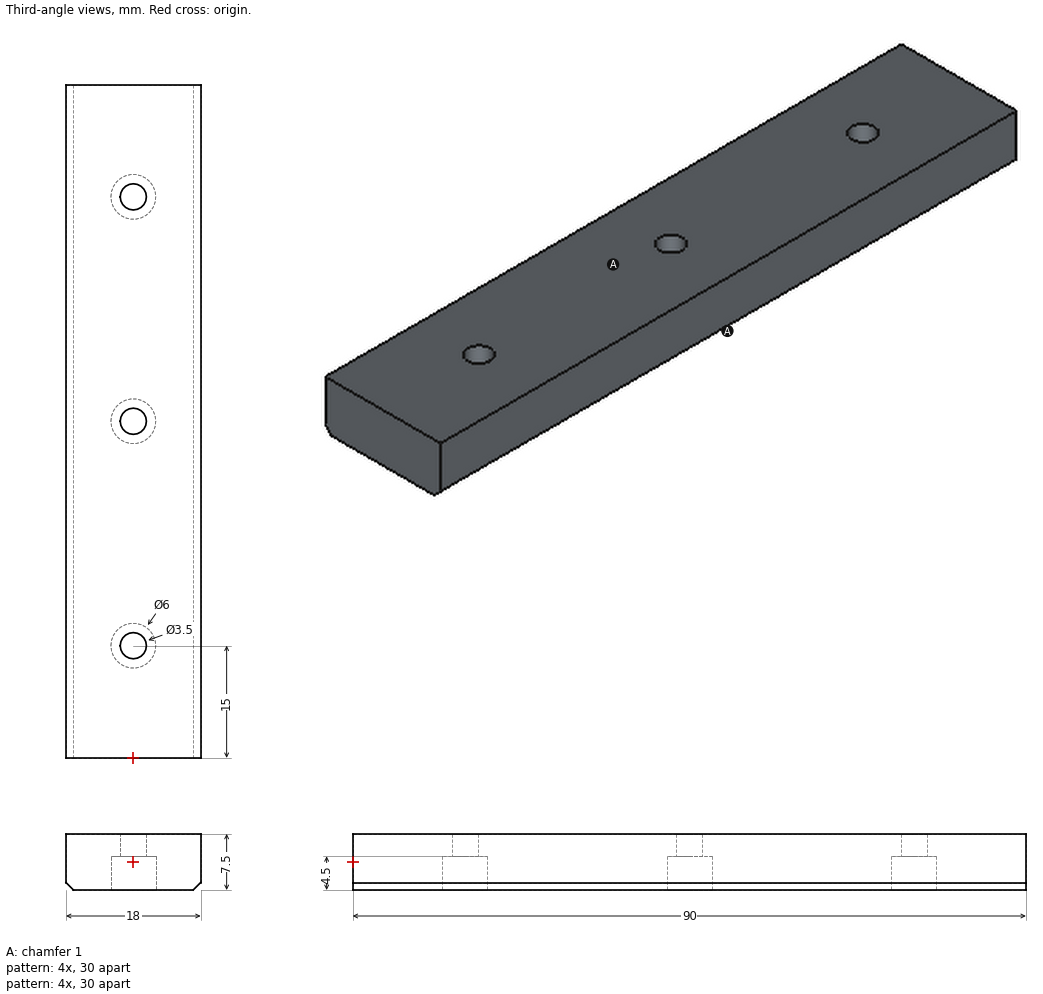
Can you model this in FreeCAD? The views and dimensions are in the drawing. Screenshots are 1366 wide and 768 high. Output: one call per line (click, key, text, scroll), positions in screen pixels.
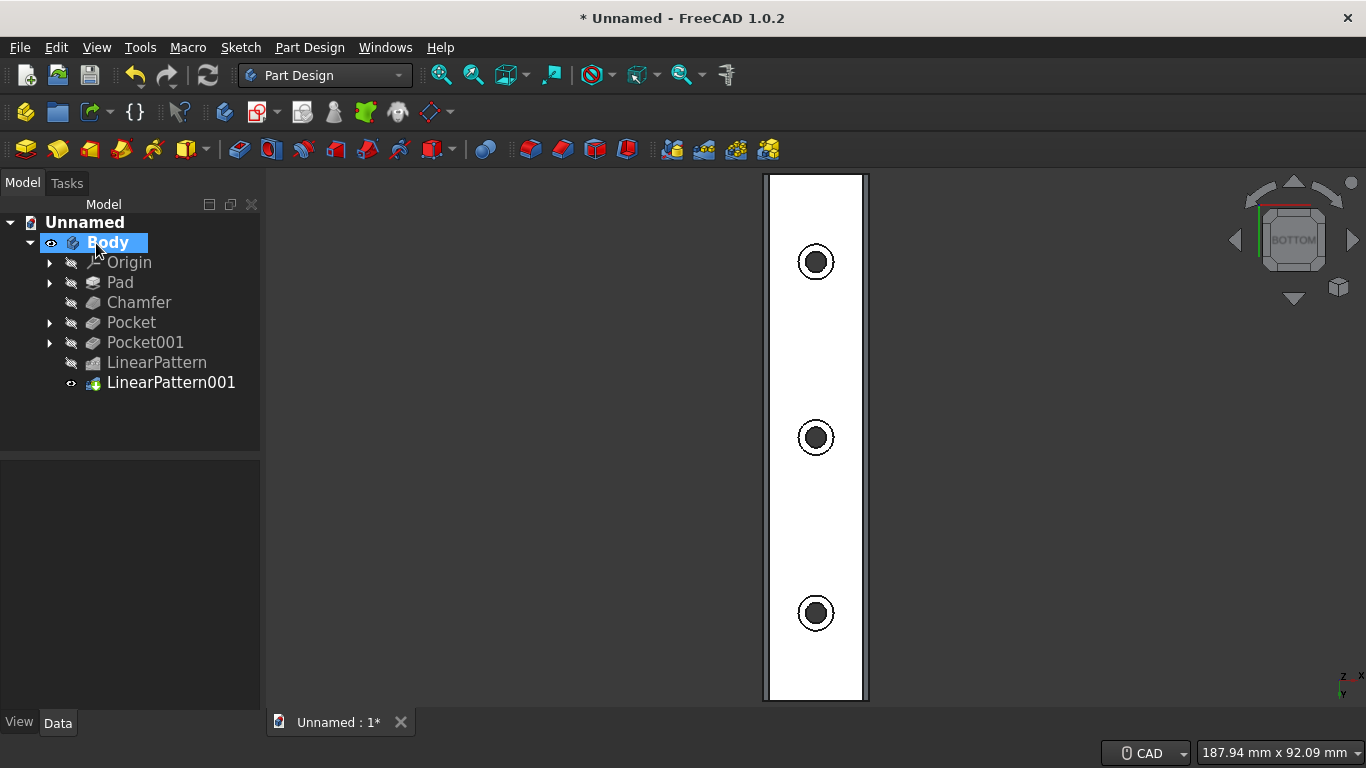
key(0)